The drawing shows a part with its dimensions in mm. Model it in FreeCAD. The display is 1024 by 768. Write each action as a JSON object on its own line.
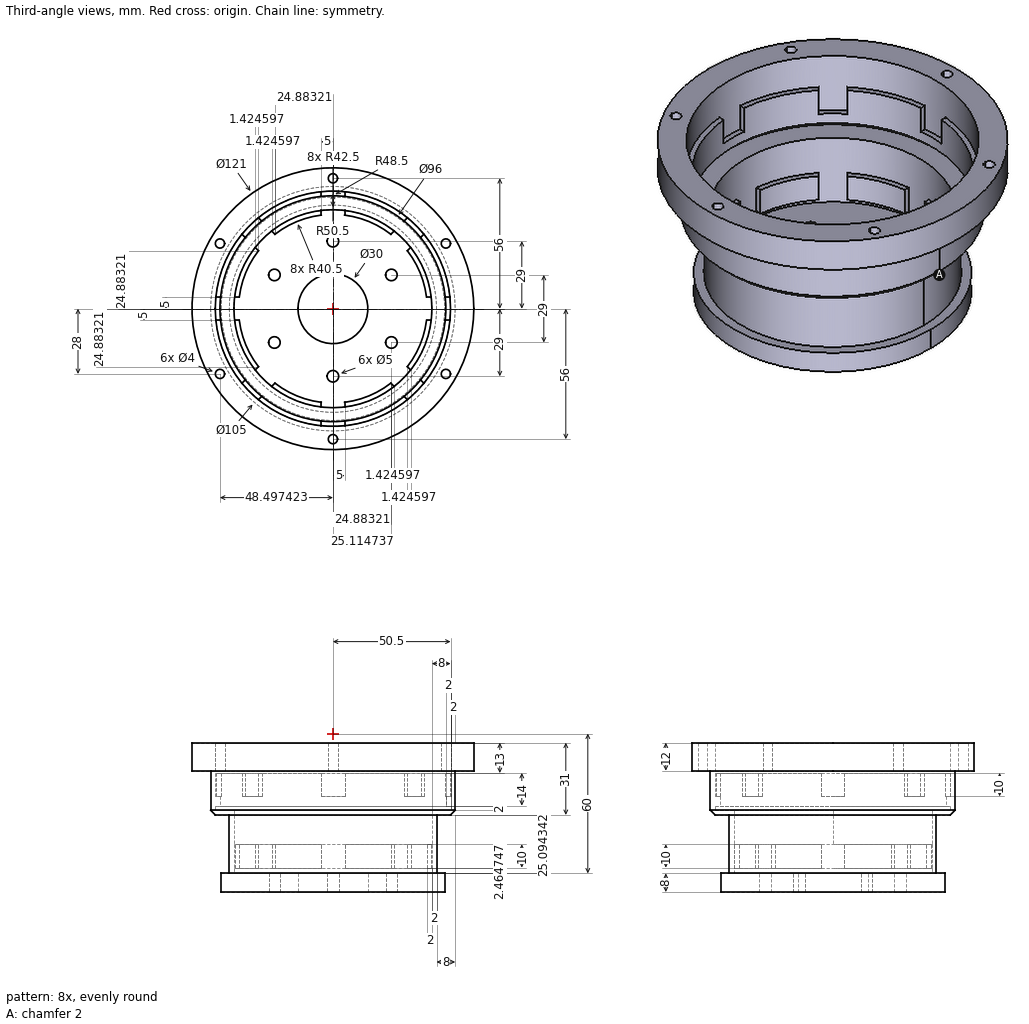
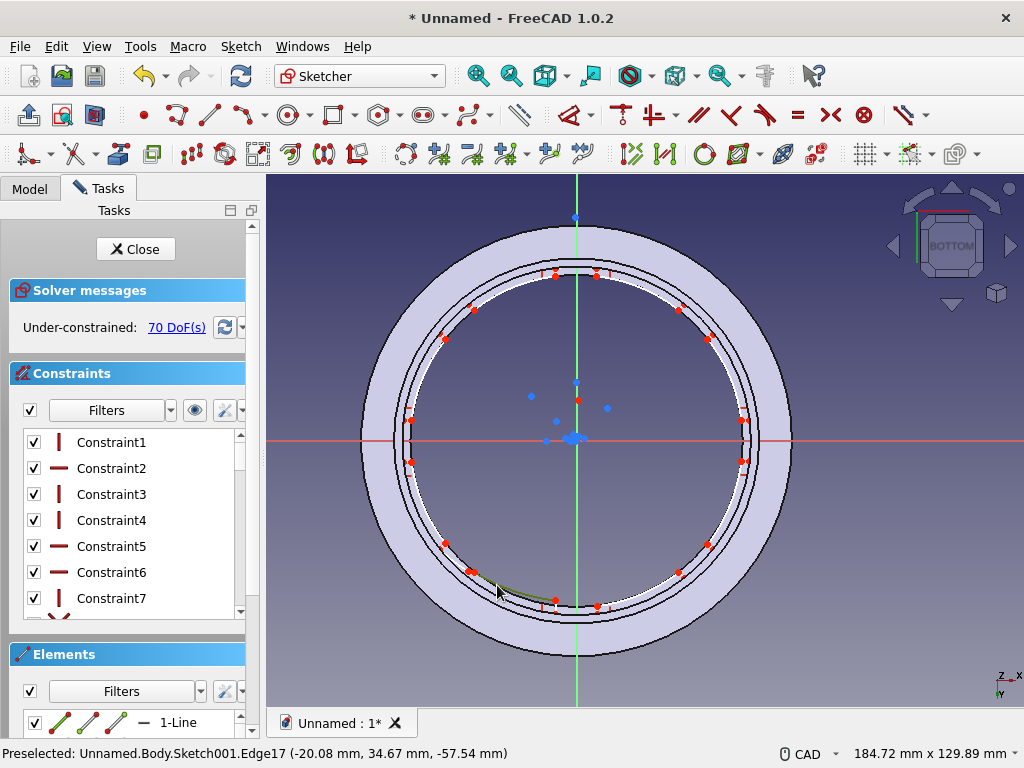
{"action": "left_click", "coordinate": [417, 488]}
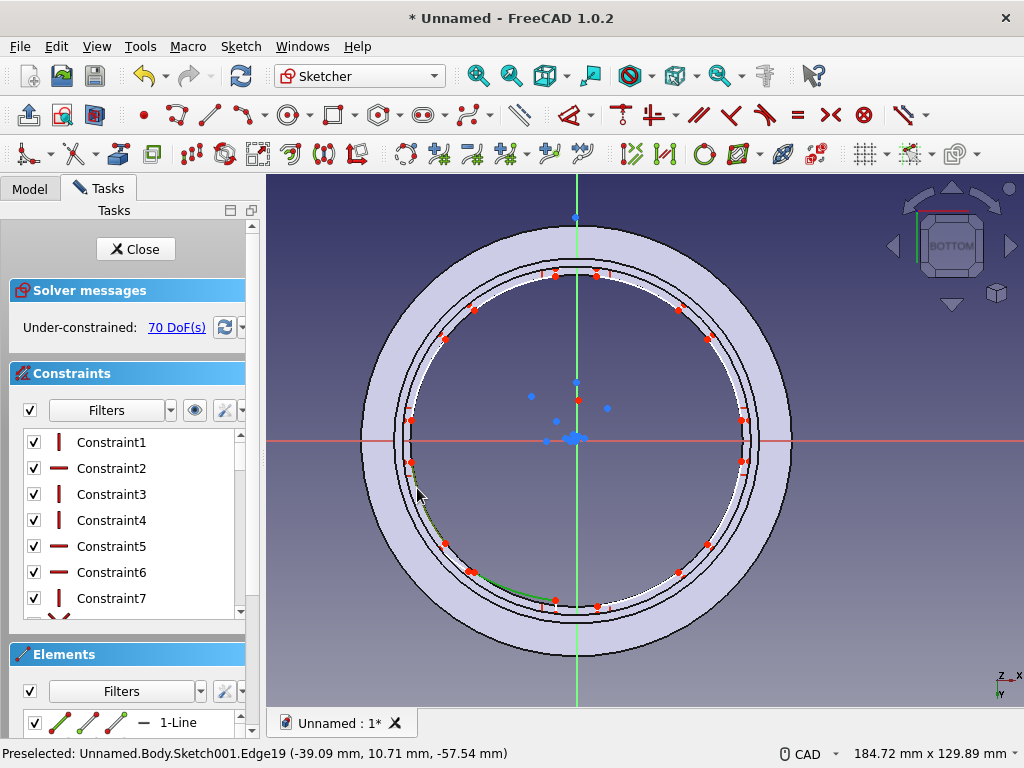
{"action": "key", "text": "c"}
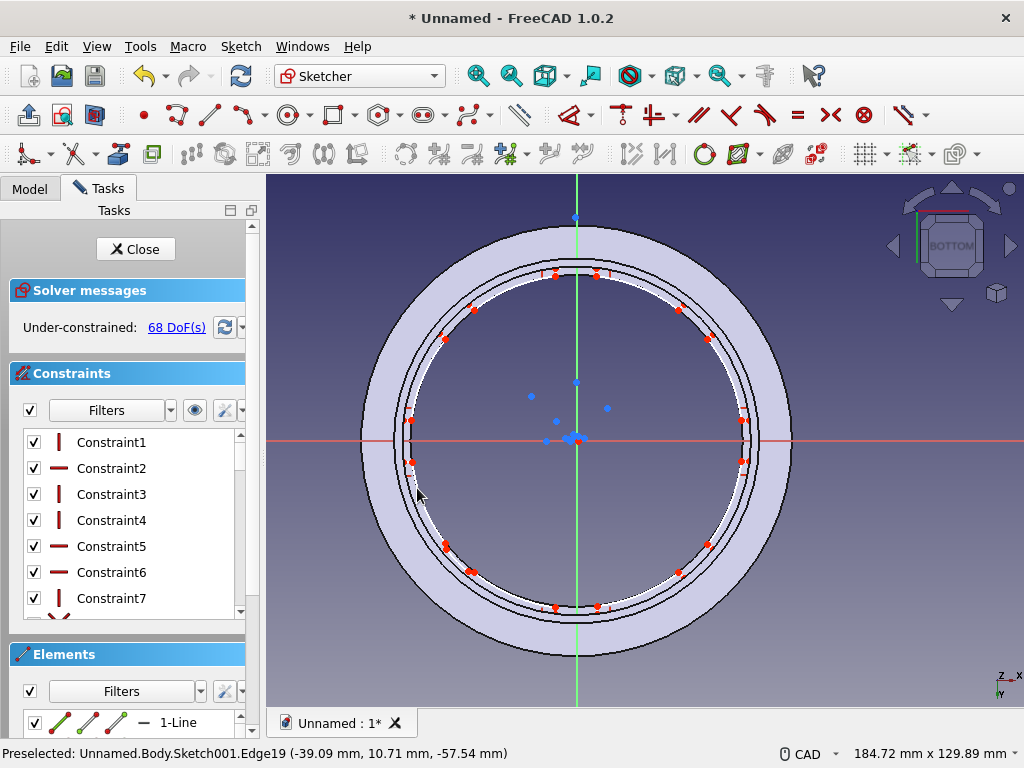
{"action": "left_click", "coordinate": [497, 588]}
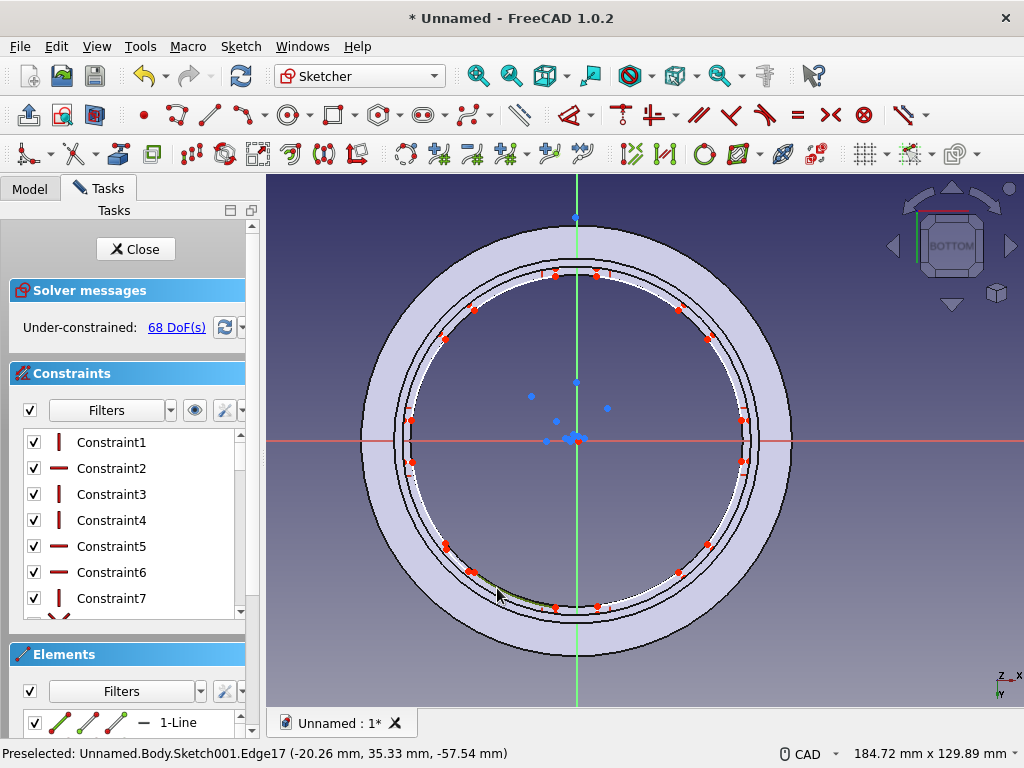
{"action": "left_click", "coordinate": [402, 441]}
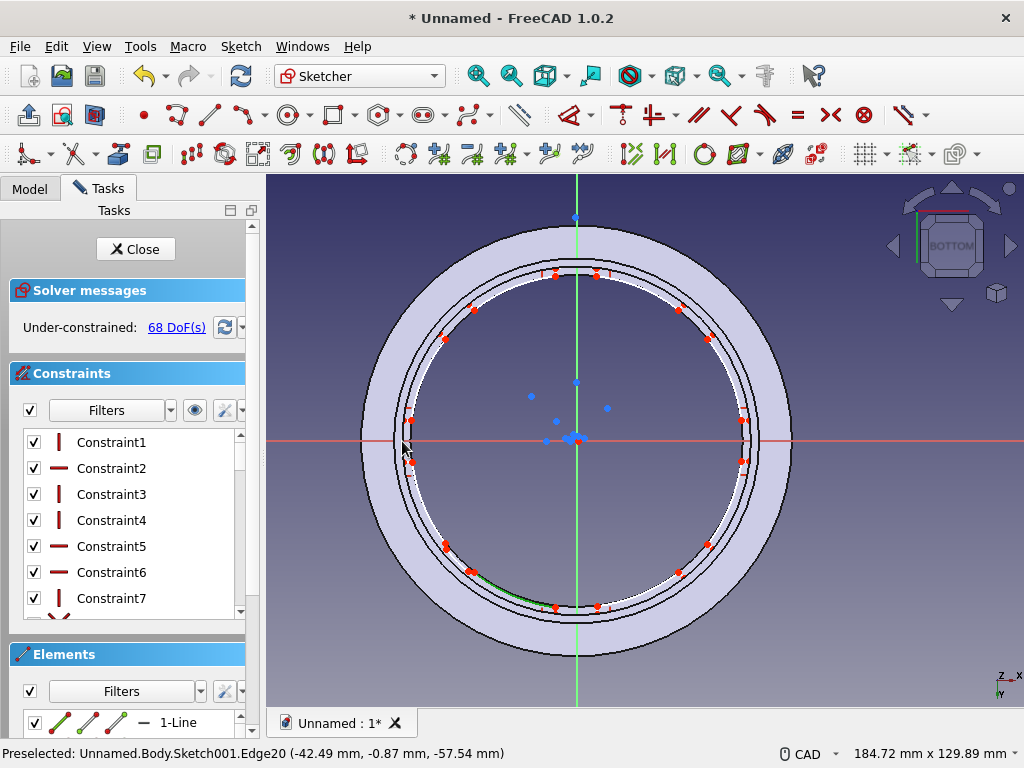
{"action": "left_click", "coordinate": [621, 116]}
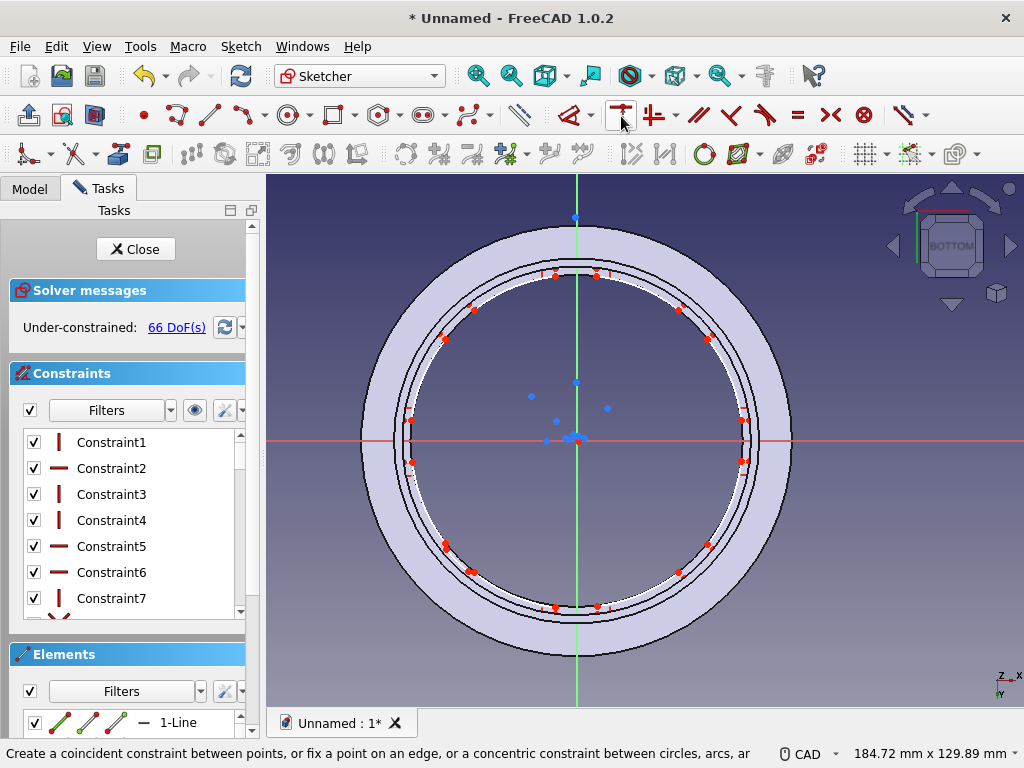
{"action": "left_click", "coordinate": [497, 588]}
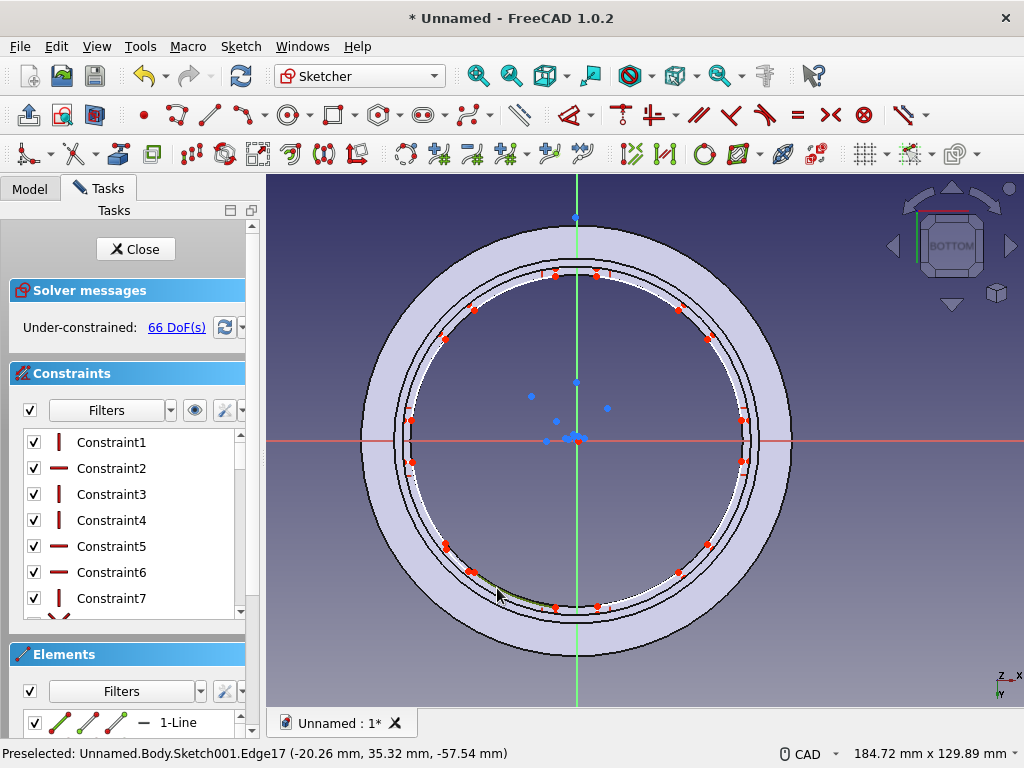
{"action": "left_click", "coordinate": [431, 362]}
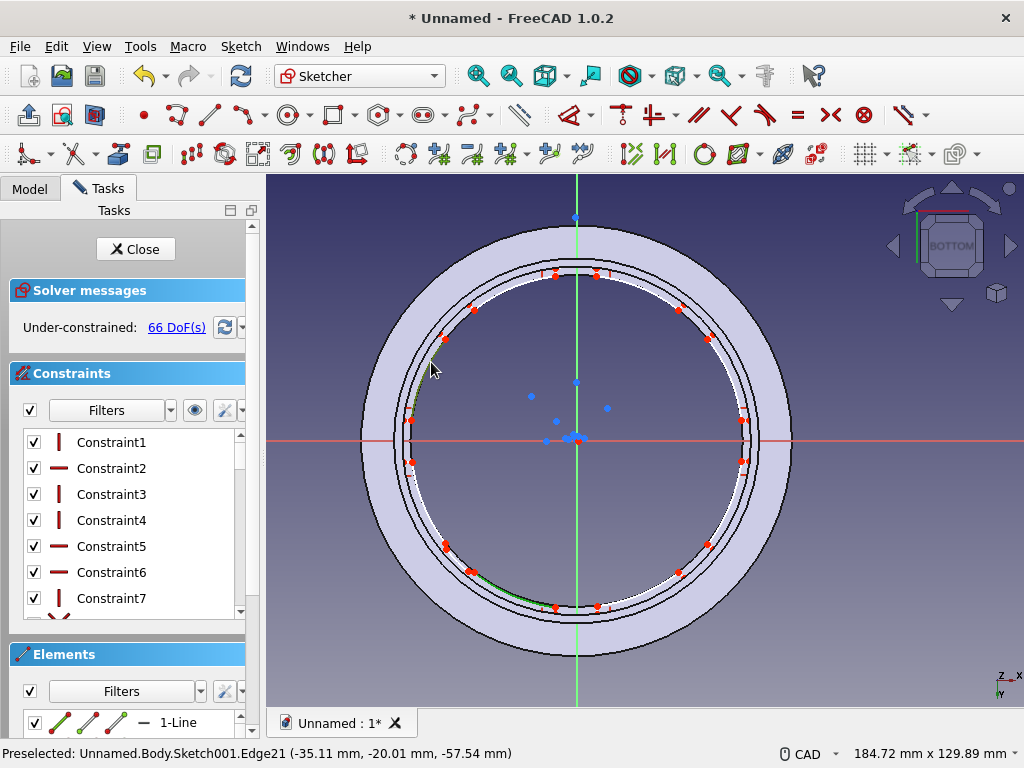
{"action": "left_click", "coordinate": [621, 116]}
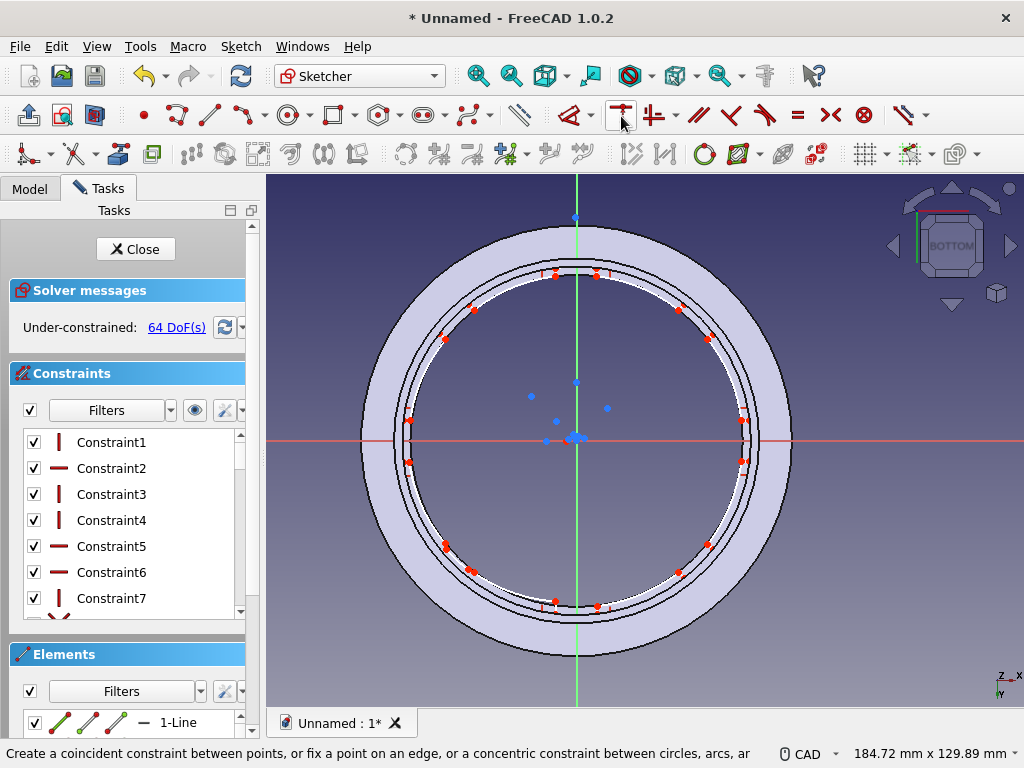
{"action": "left_click", "coordinate": [497, 586]}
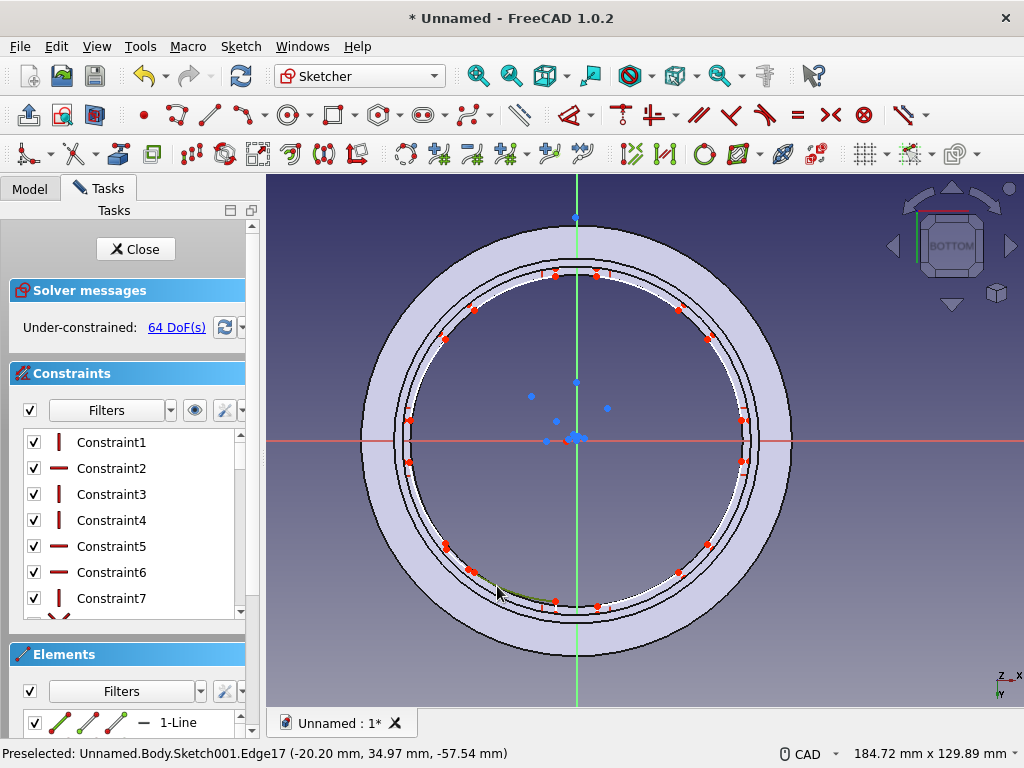
{"action": "left_click", "coordinate": [459, 312]}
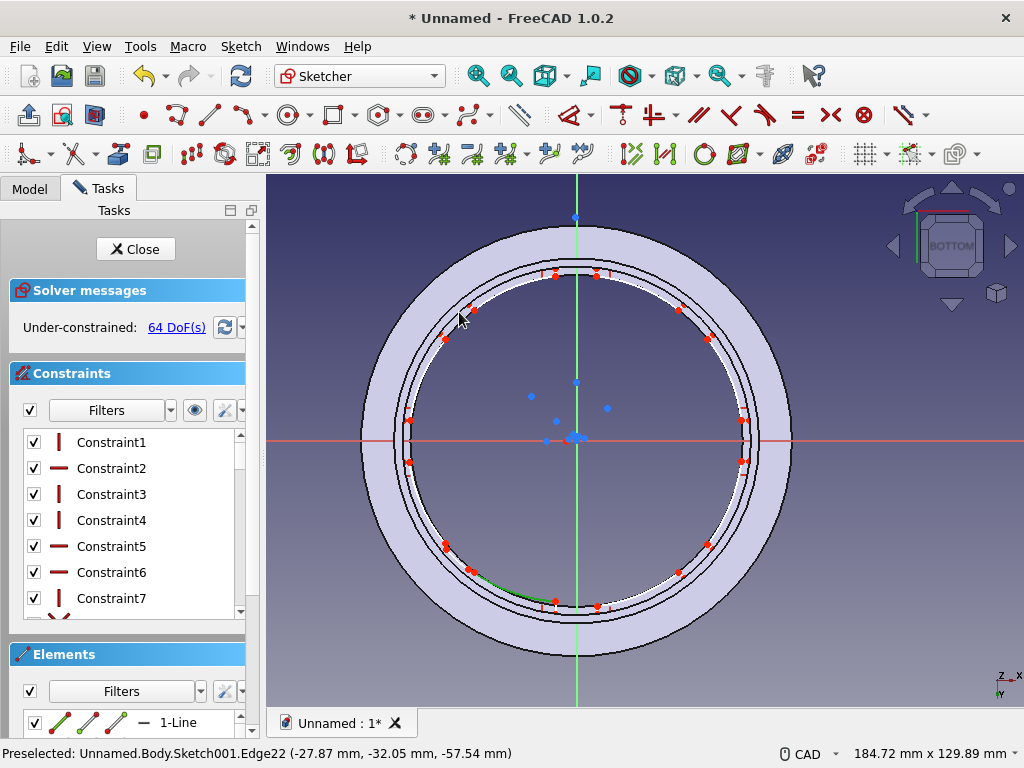
{"action": "key", "text": "c"}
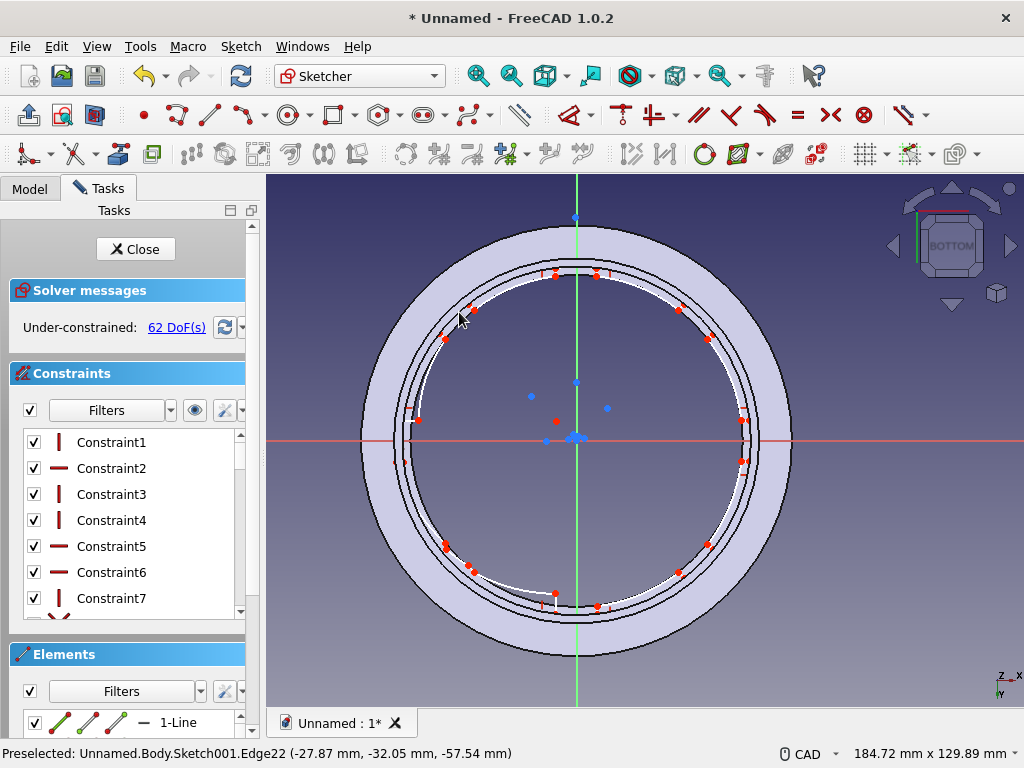
{"action": "left_click", "coordinate": [497, 583]}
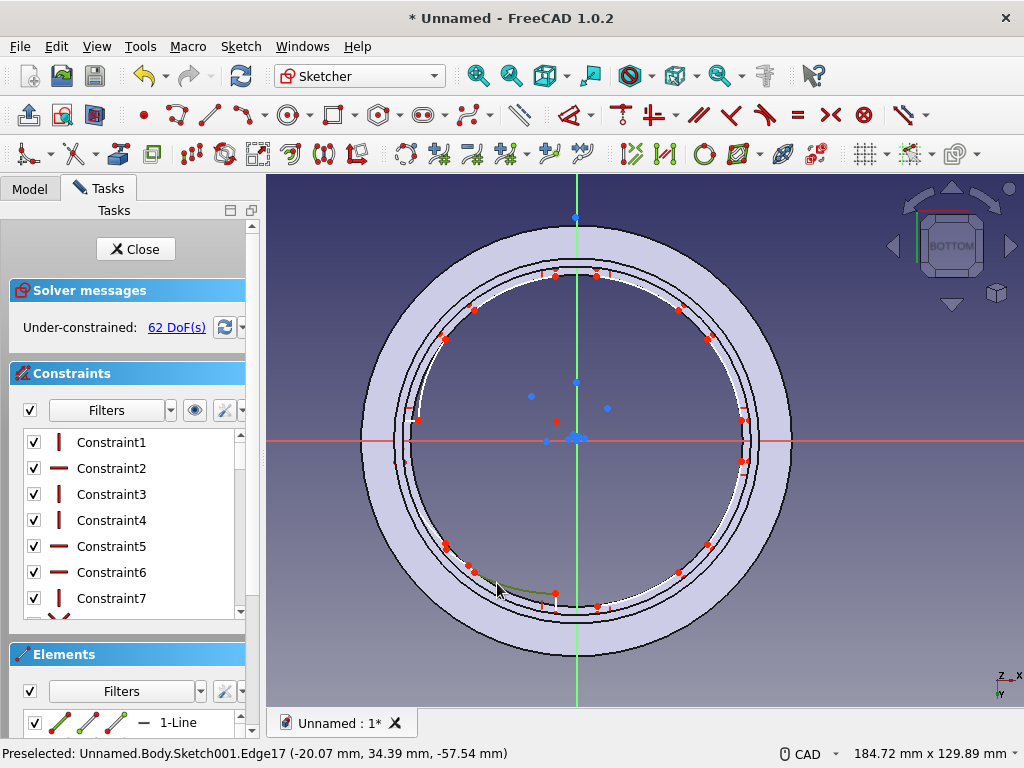
{"action": "left_click", "coordinate": [530, 282]}